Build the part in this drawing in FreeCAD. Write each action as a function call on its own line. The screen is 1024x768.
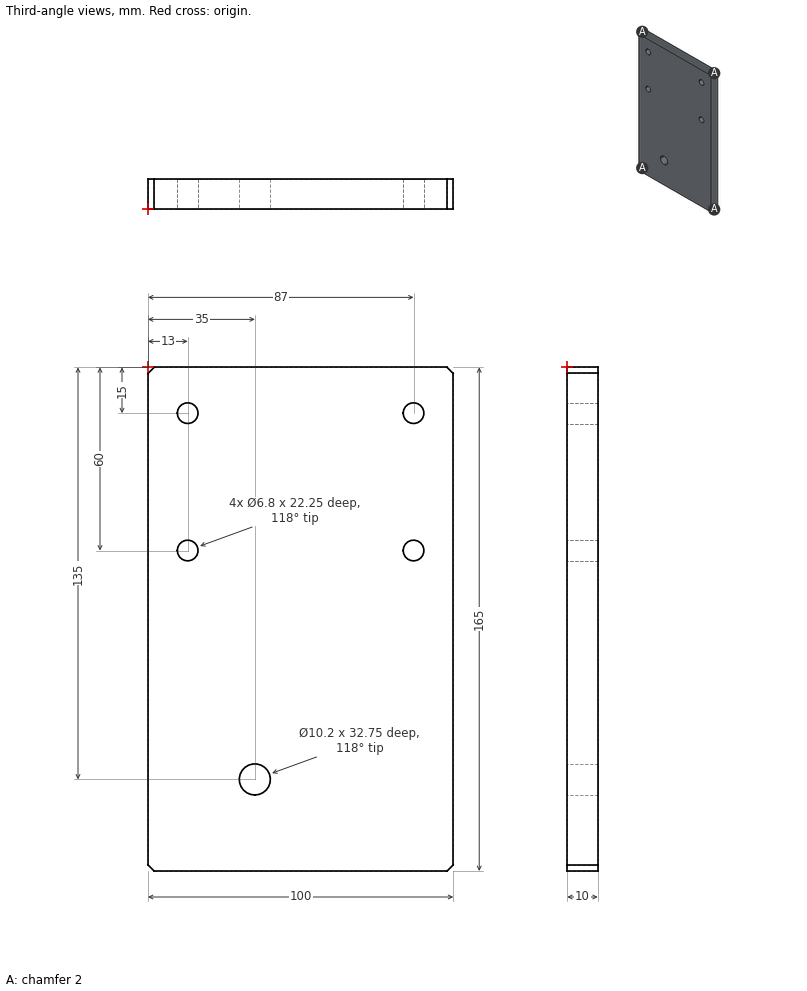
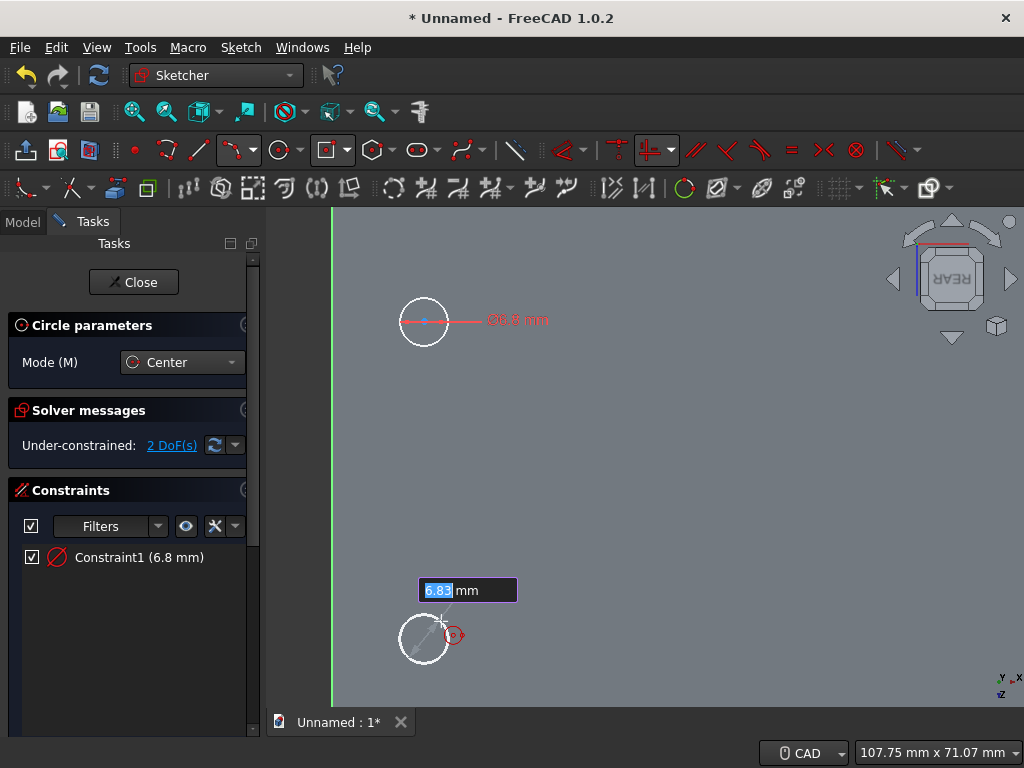
text(6.8)
key(Return)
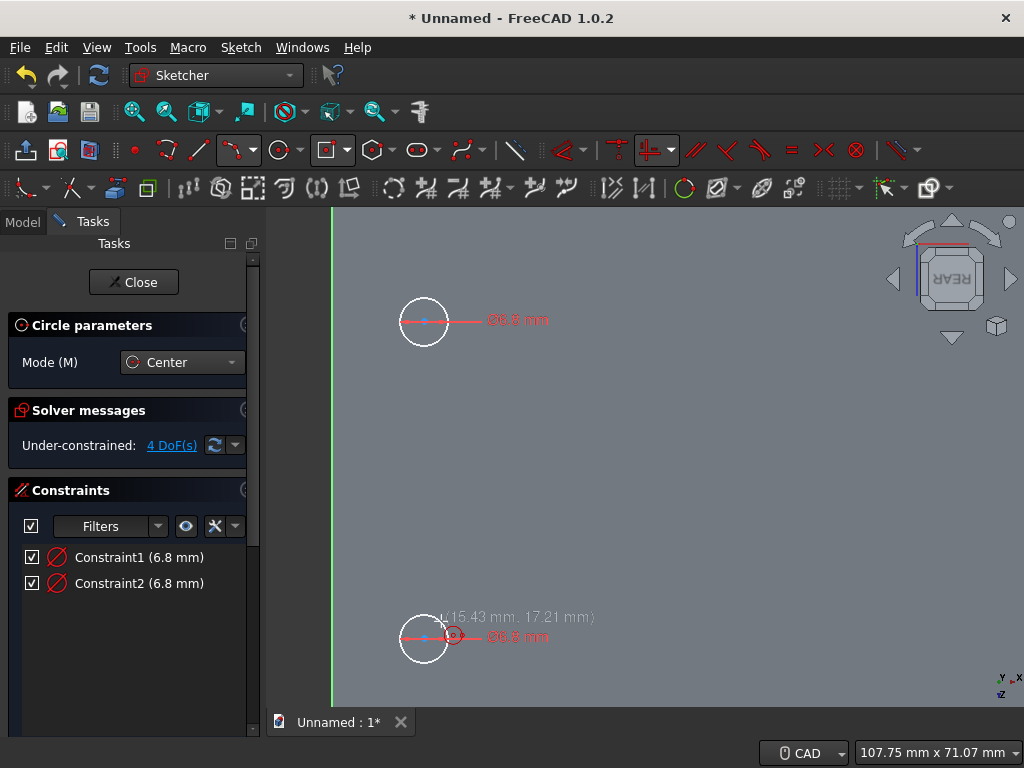
scroll(426, 329, down, 2)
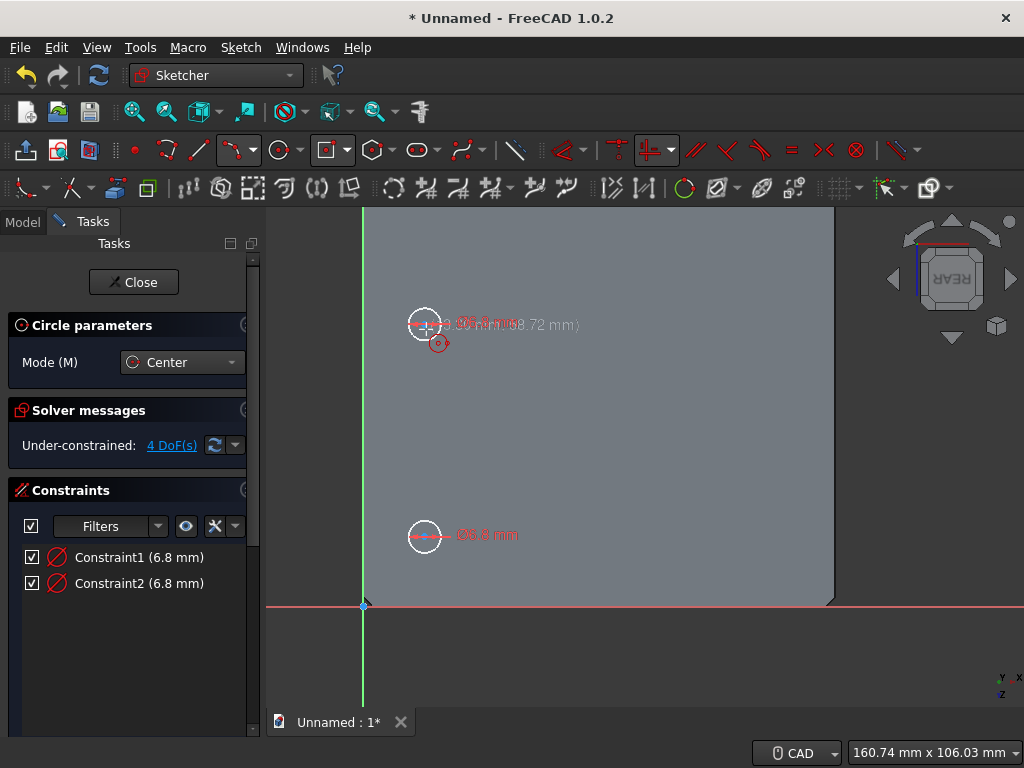
scroll(774, 536, up, 2)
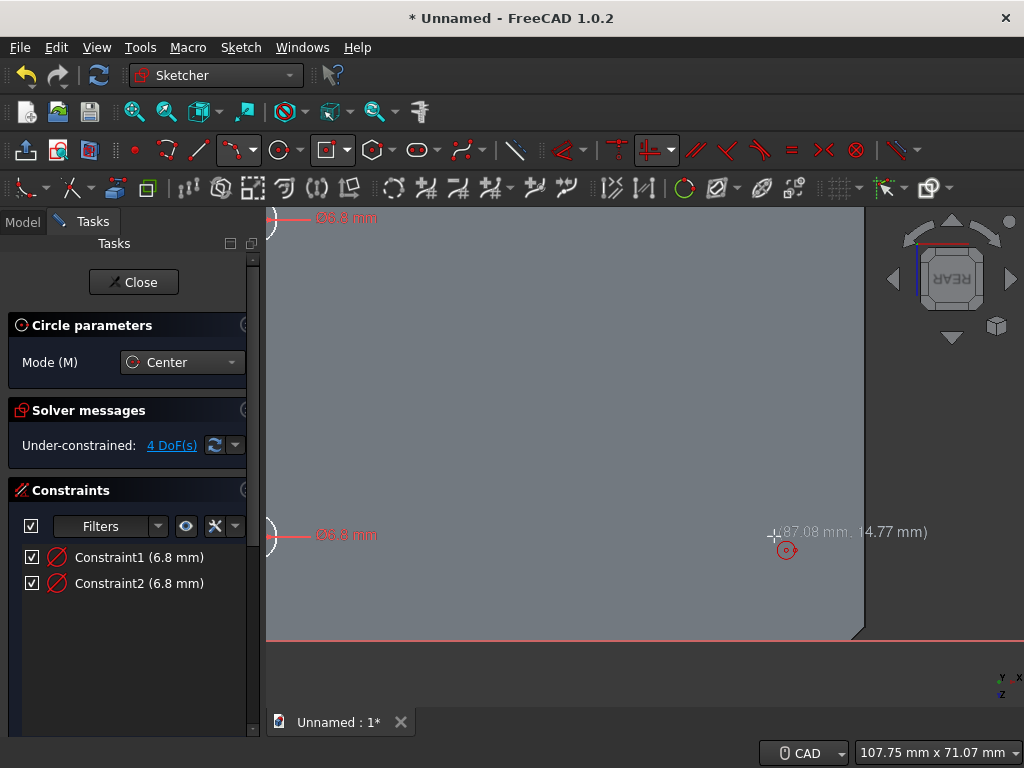
click(773, 536)
move(790, 519)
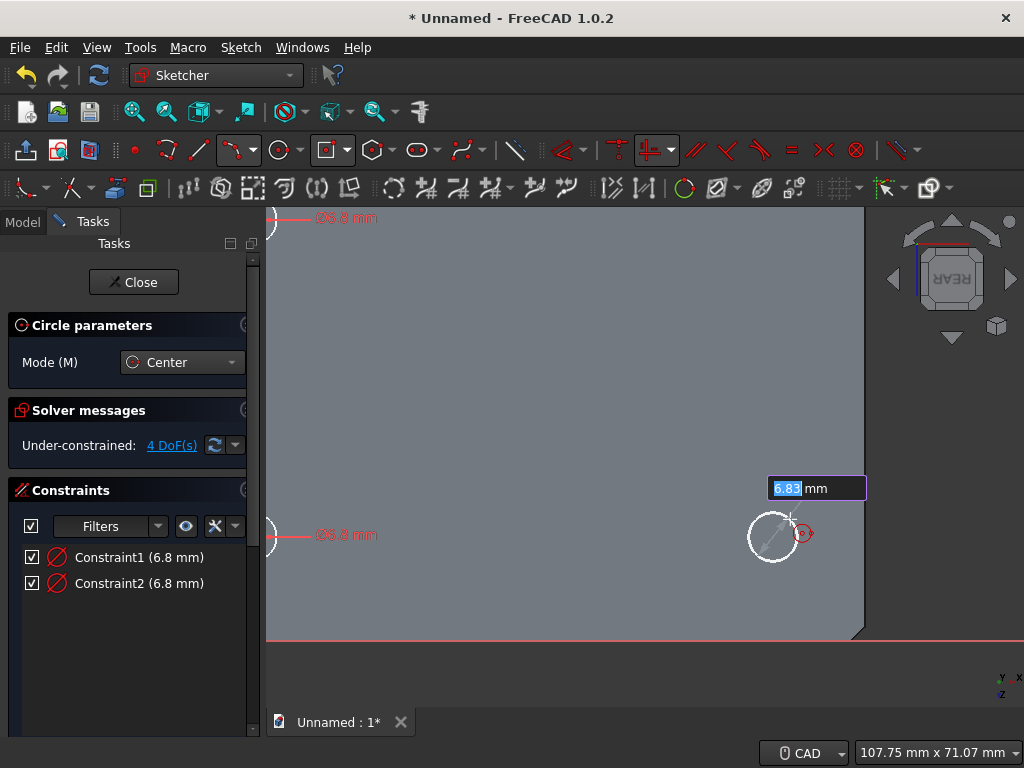
text(6.8)
key(Return)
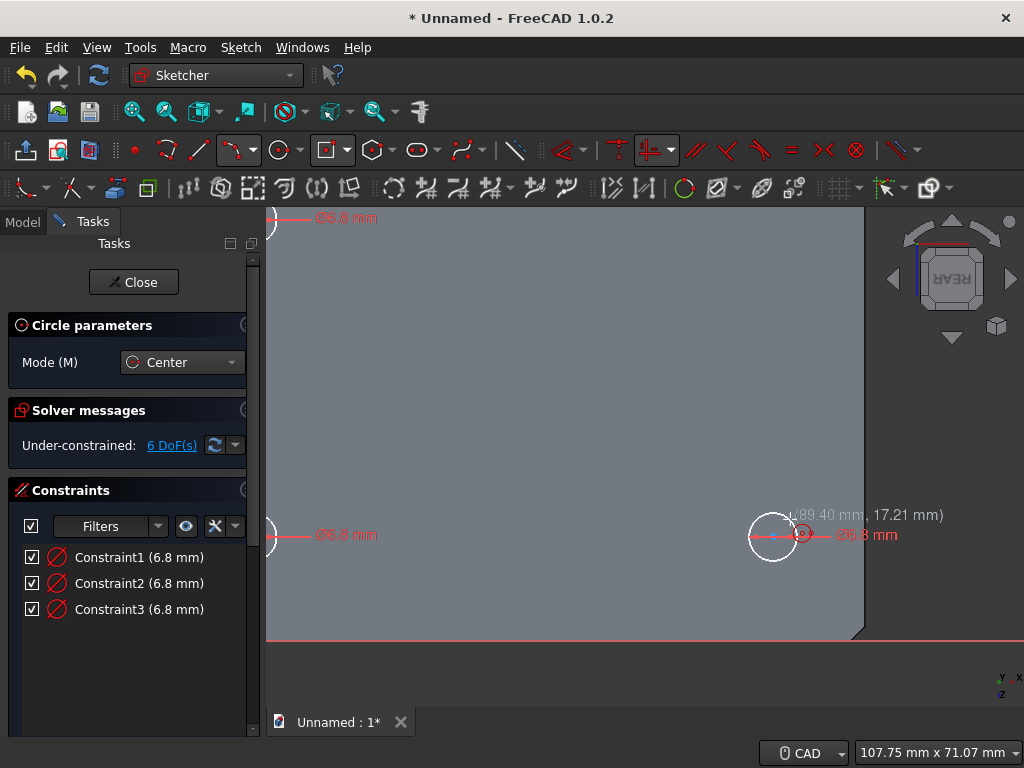
scroll(775, 536, down, 2)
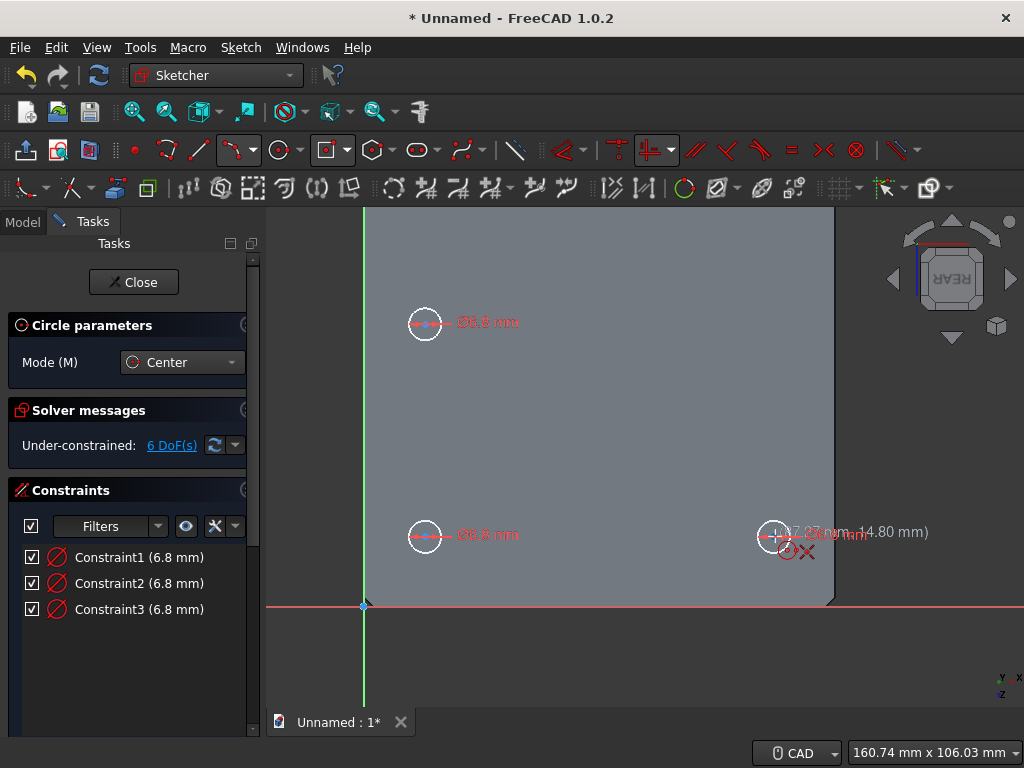
scroll(774, 324, up, 2)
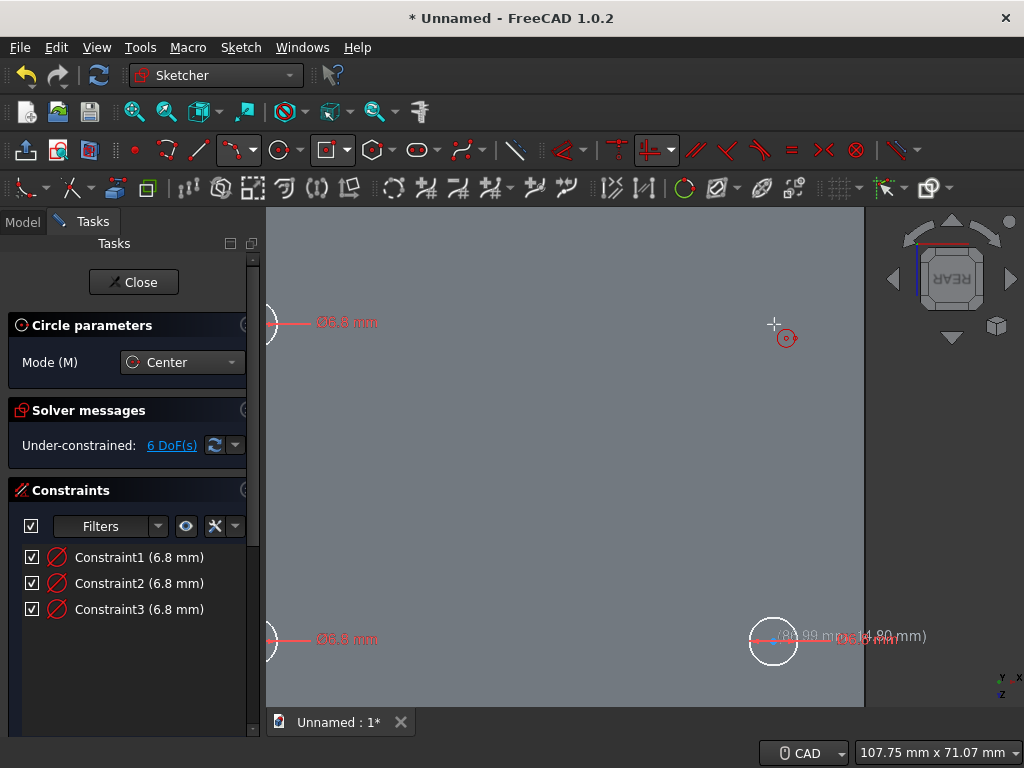
click(774, 323)
move(791, 307)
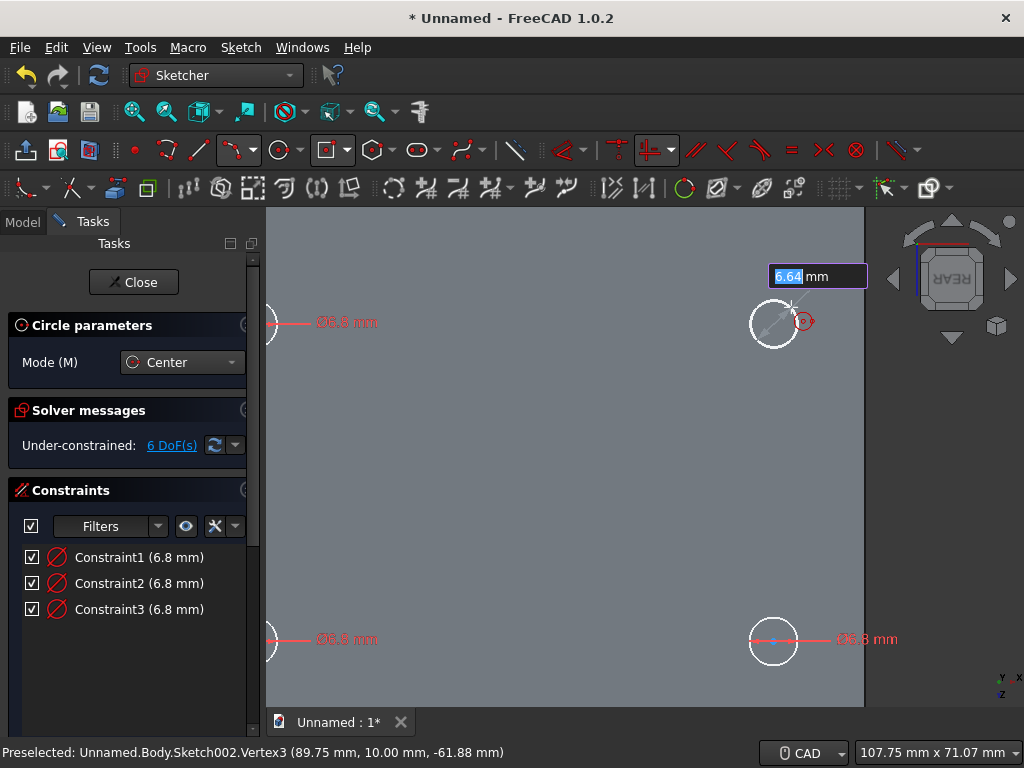
text(6.8)
key(Return)
key(Escape)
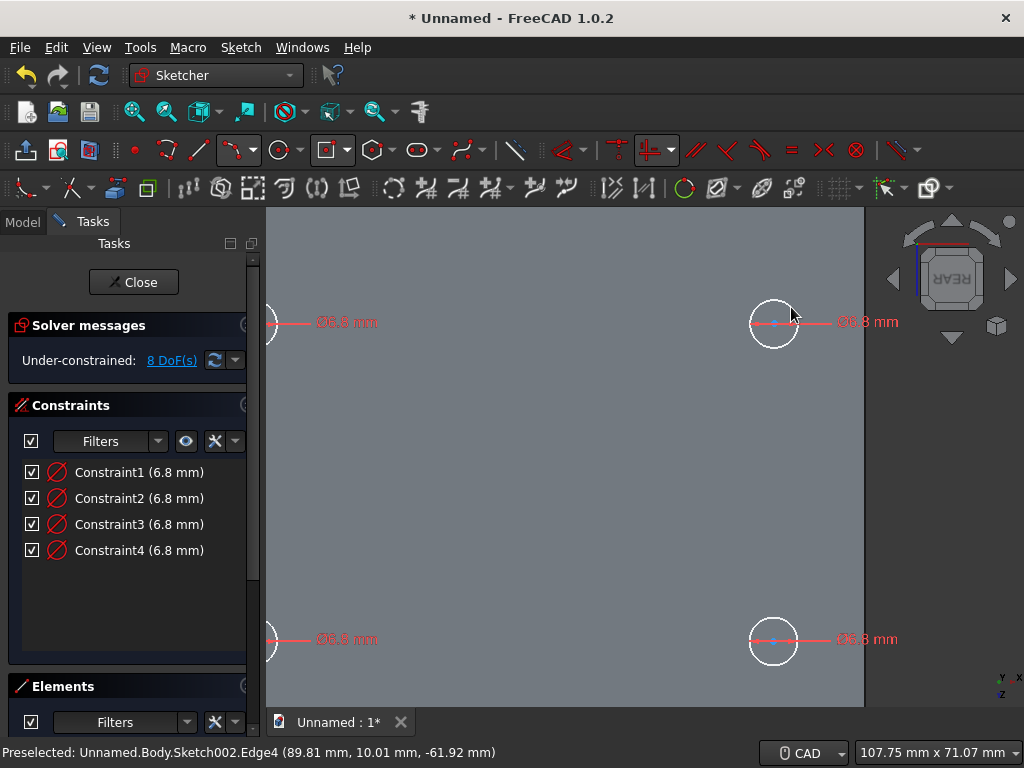
scroll(774, 324, down, 2)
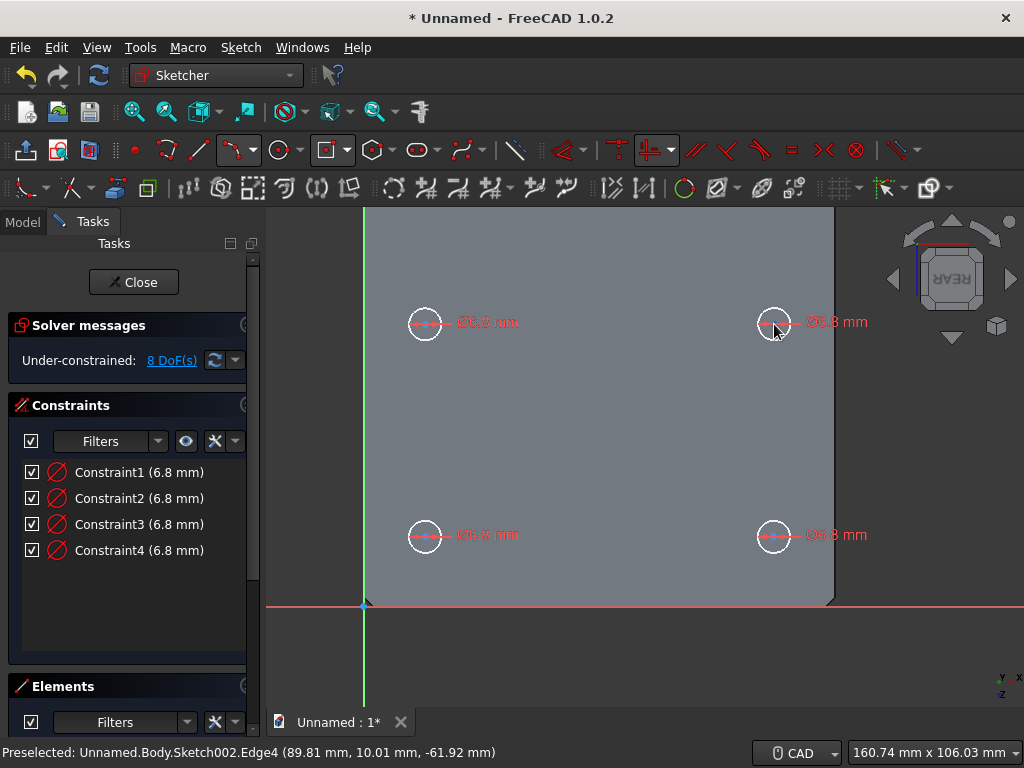
click(425, 324)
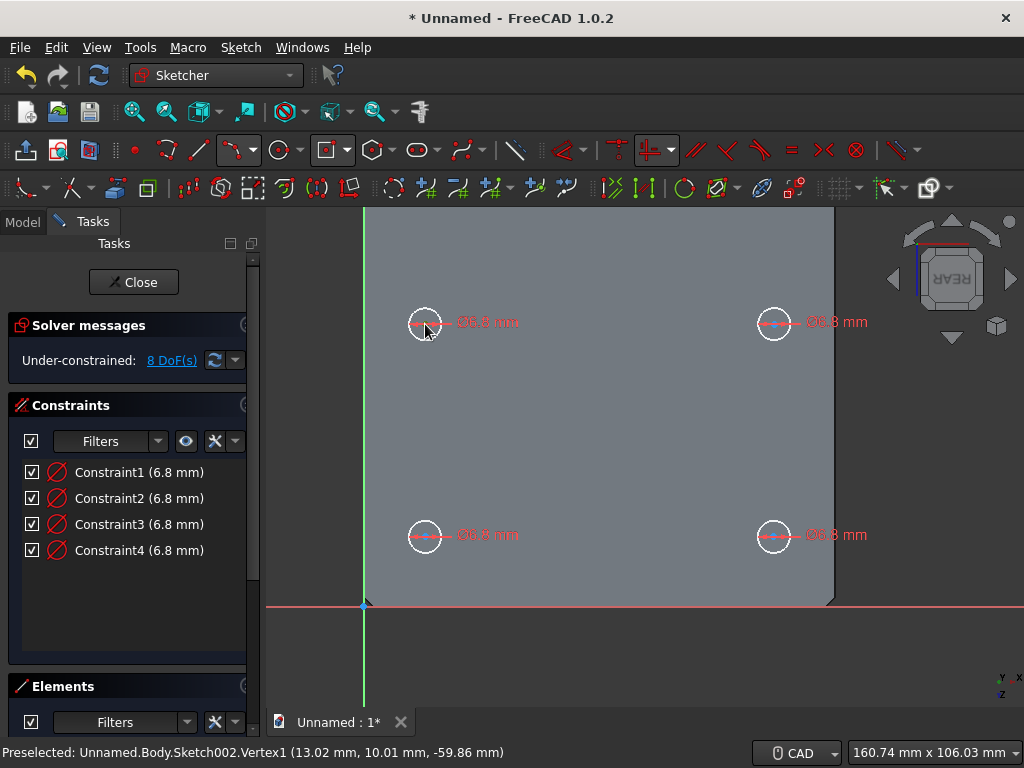
click(586, 150)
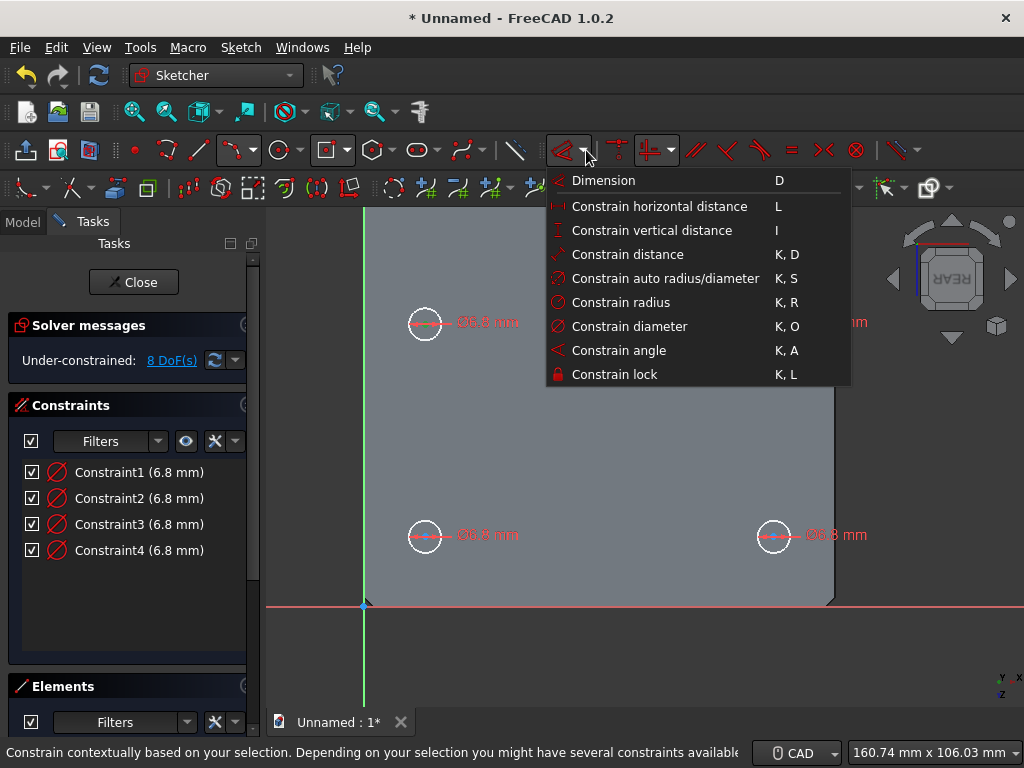
click(699, 206)